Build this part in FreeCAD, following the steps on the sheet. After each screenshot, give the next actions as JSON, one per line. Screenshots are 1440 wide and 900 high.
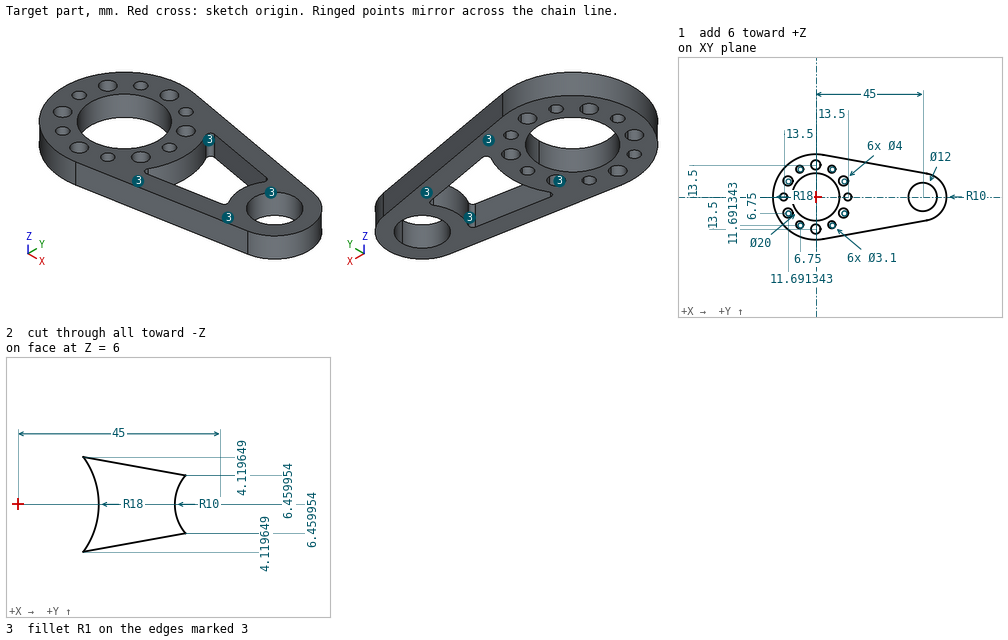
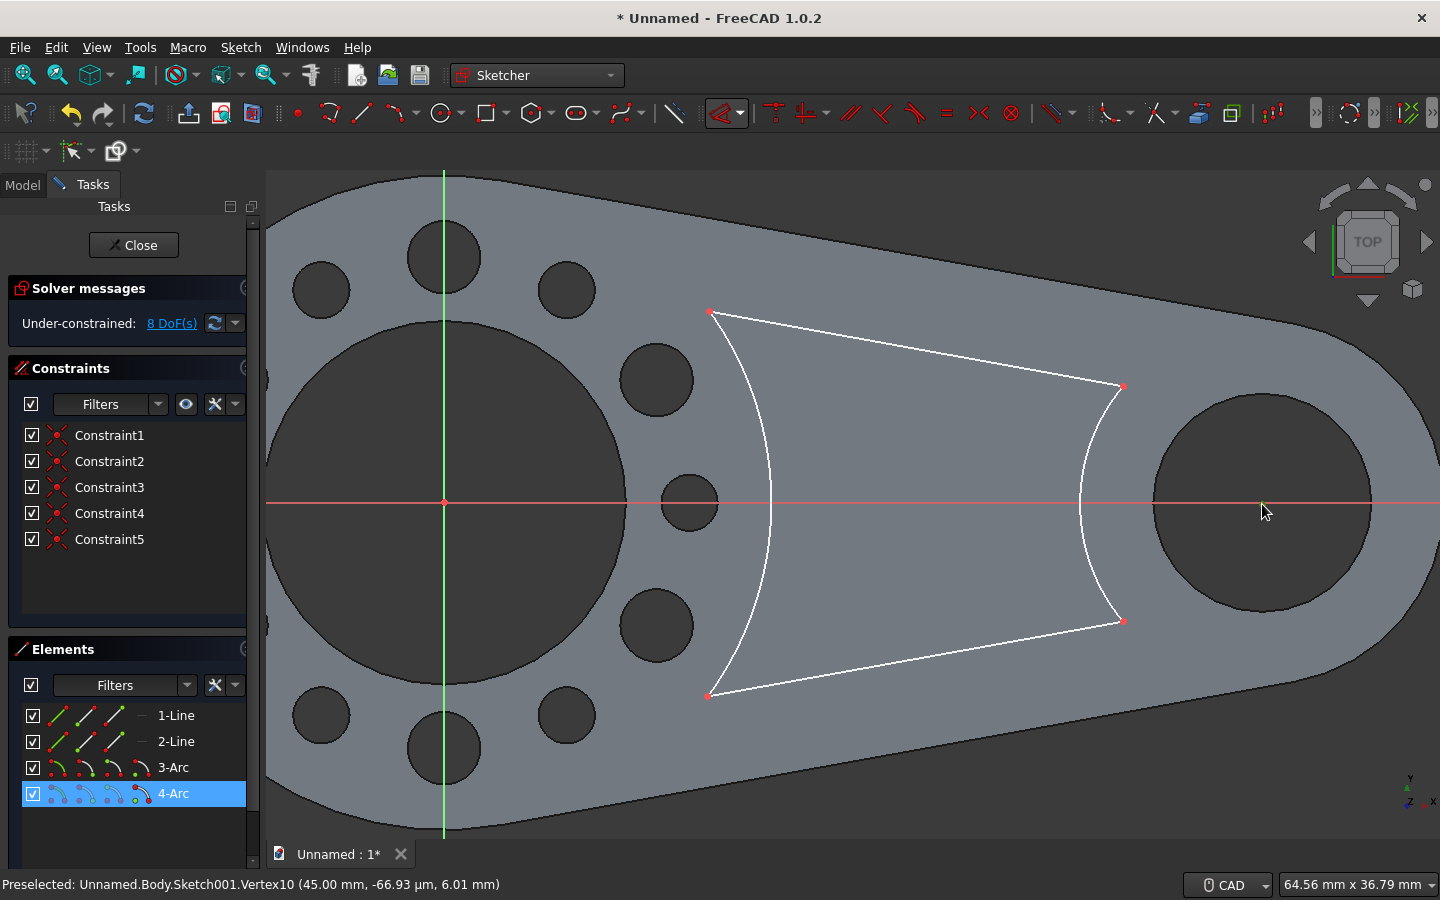
{"action": "left_click", "coordinate": [364, 503]}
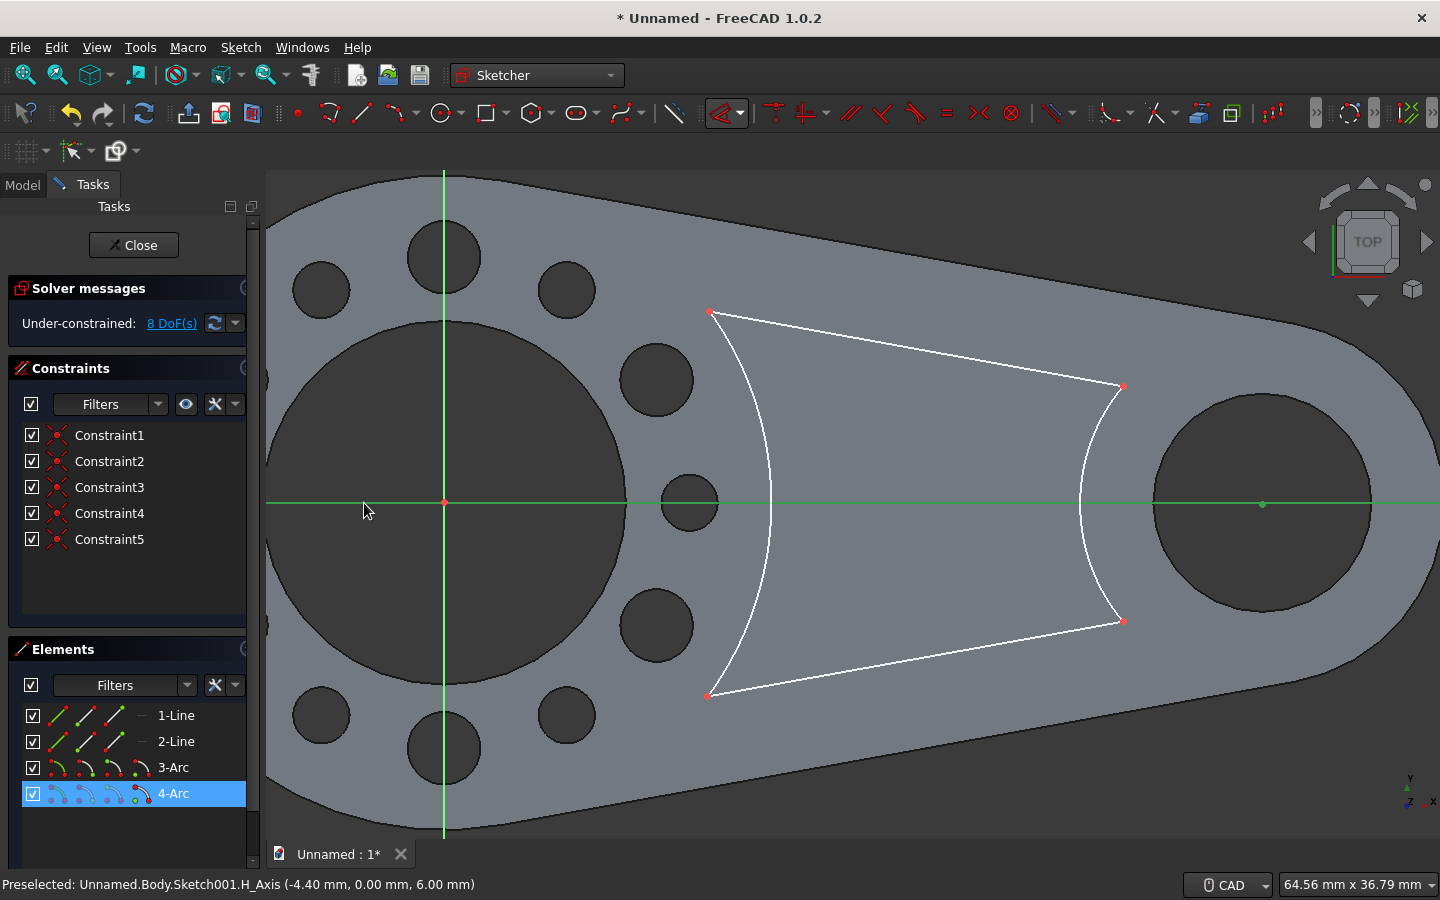
{"action": "key", "text": "c"}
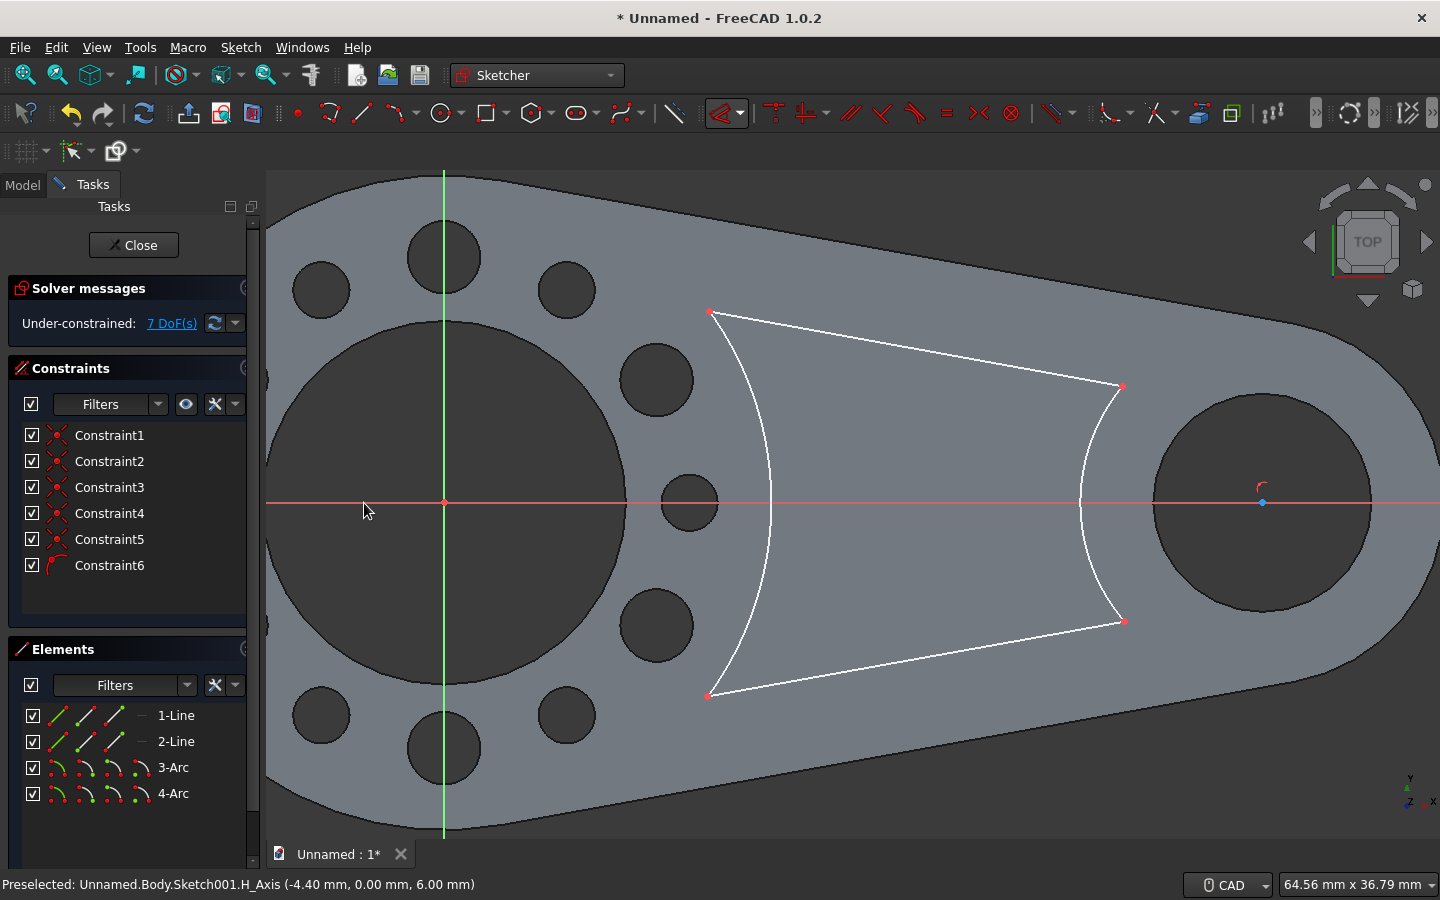
{"action": "left_click", "coordinate": [720, 114]}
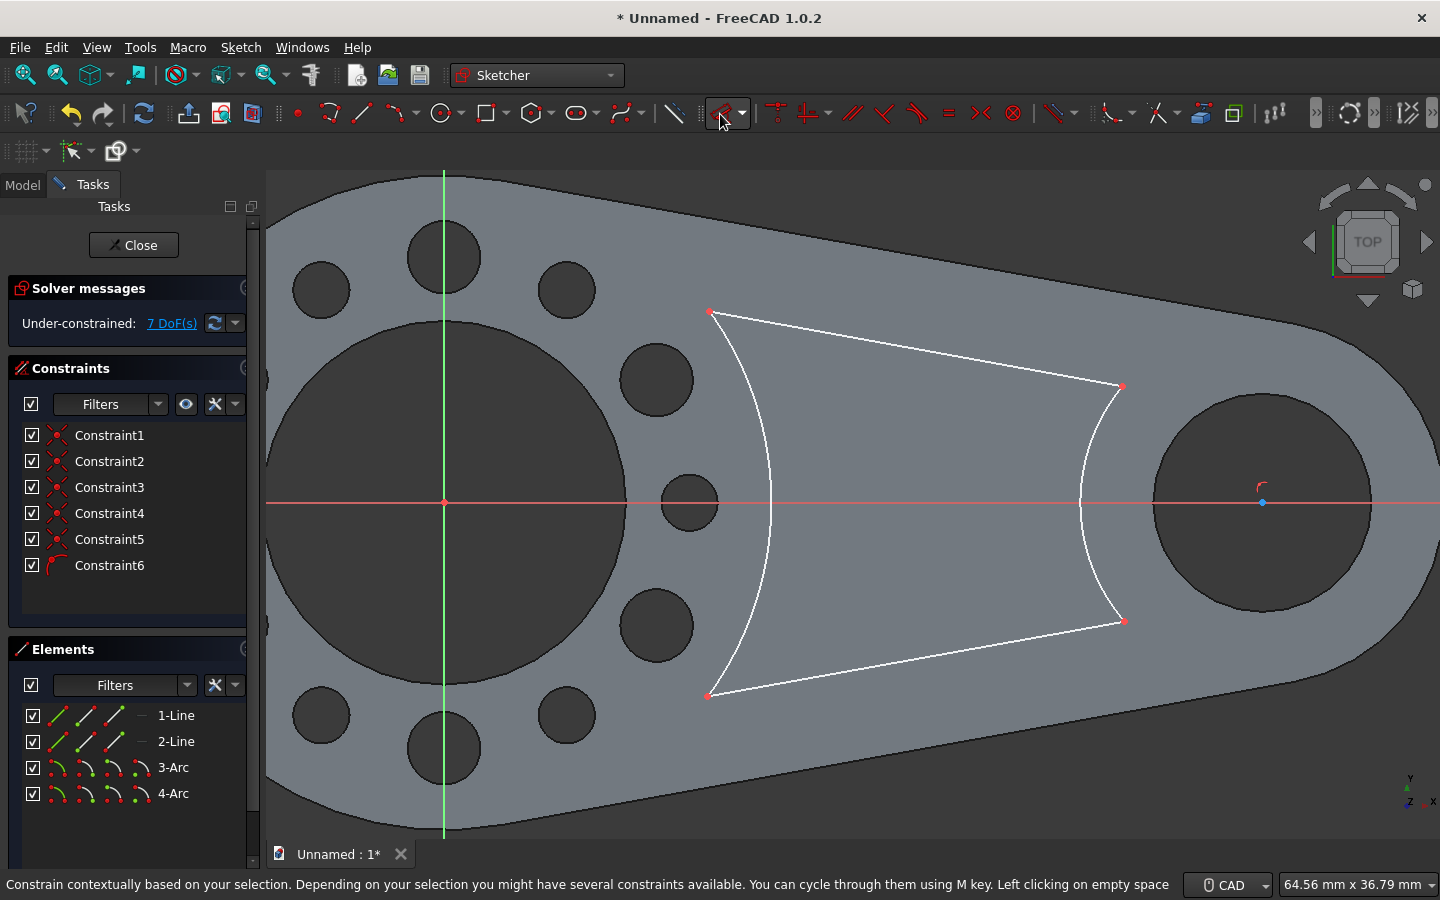
{"action": "left_click", "coordinate": [761, 586]}
{"action": "left_click", "coordinate": [792, 594]}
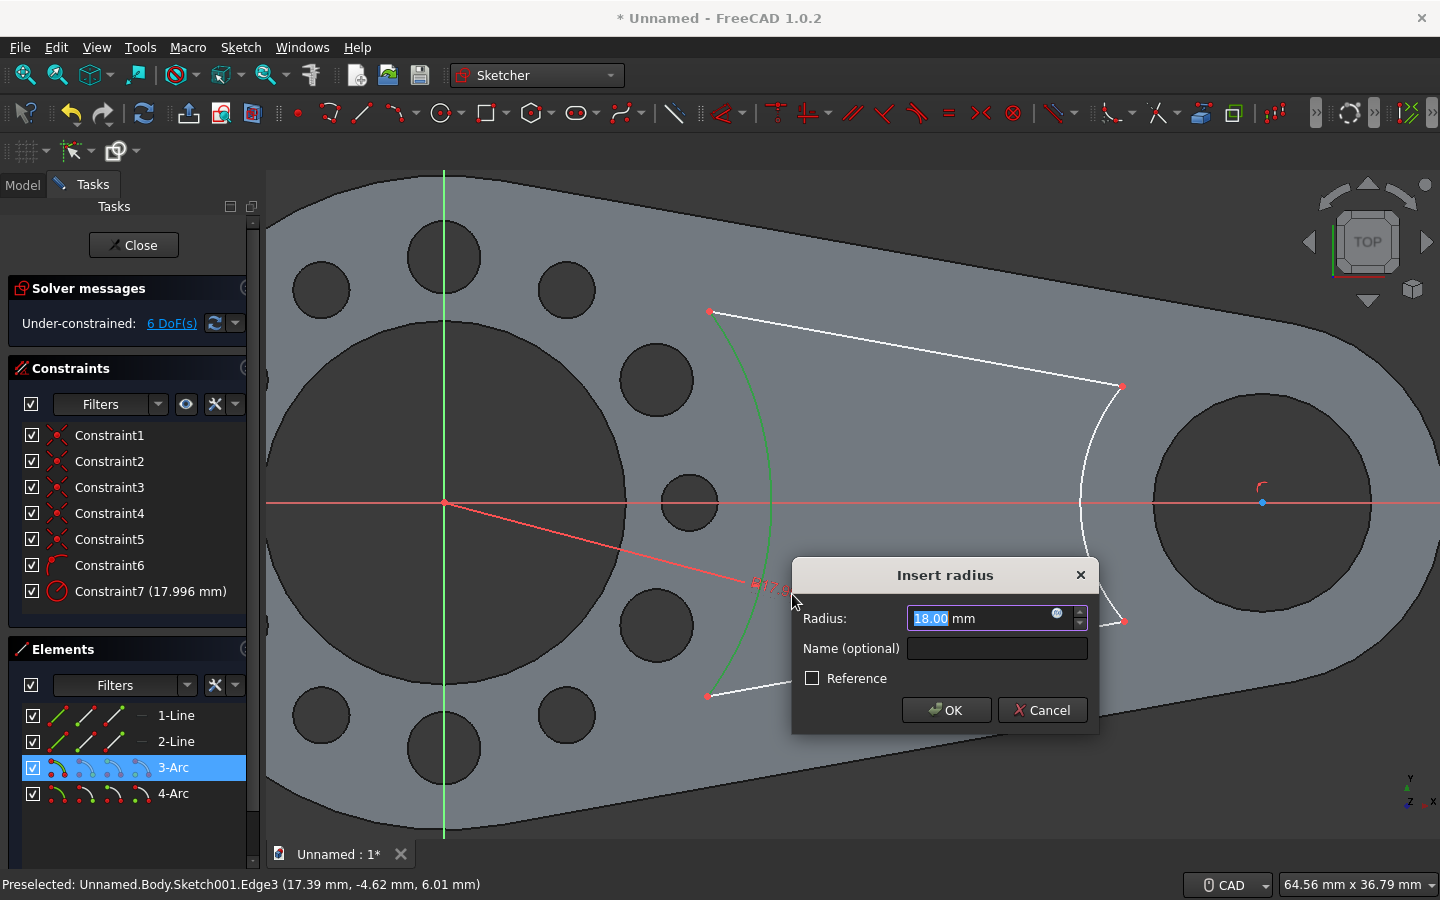
{"action": "type", "text": "18"}
{"action": "key", "text": "Return"}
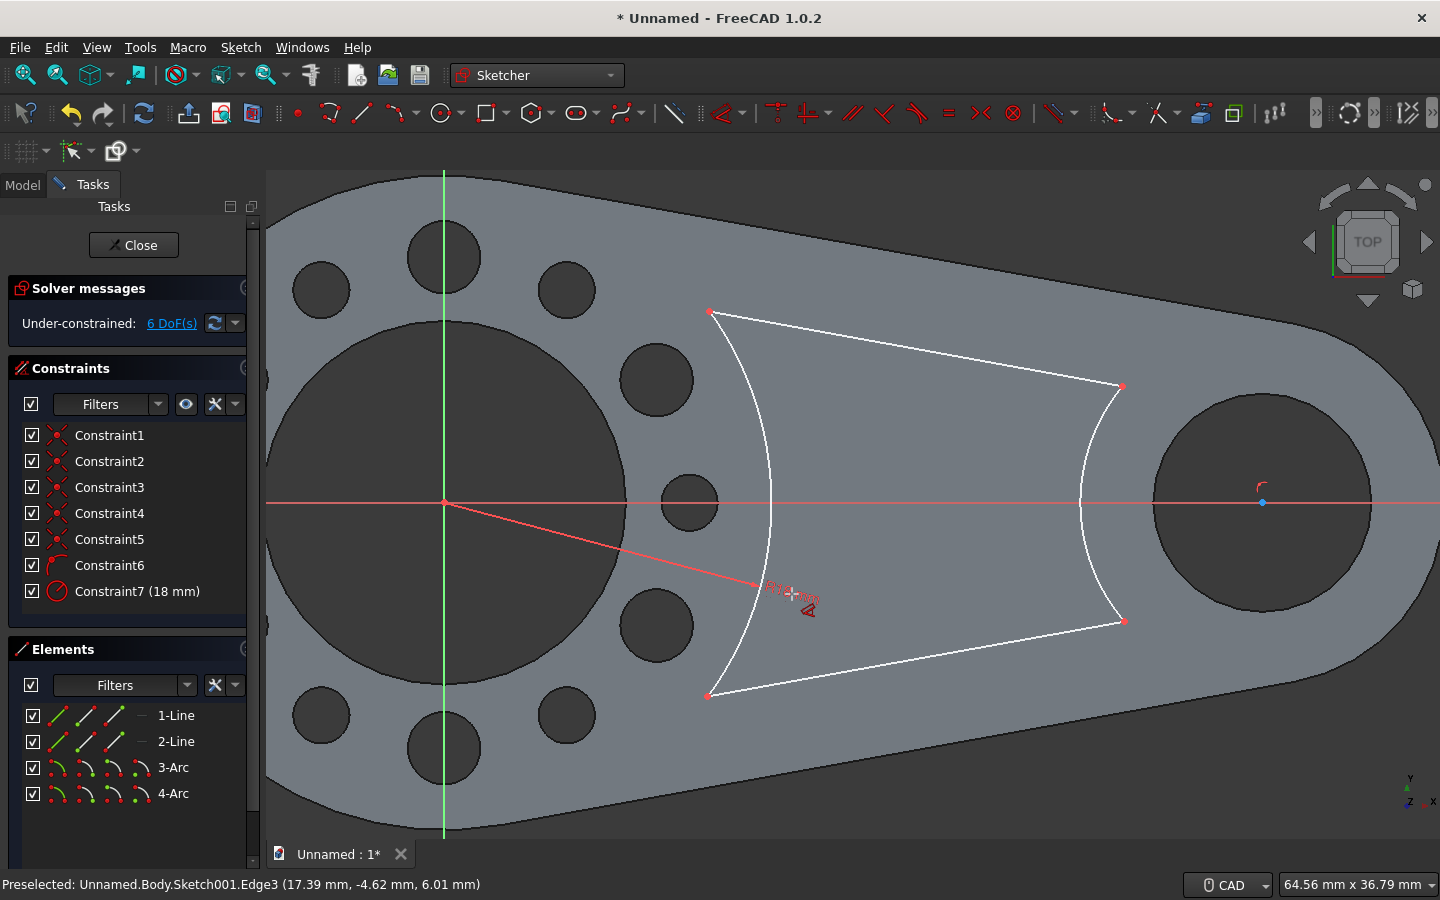
{"action": "left_click", "coordinate": [1087, 454]}
{"action": "left_click", "coordinate": [1056, 445]}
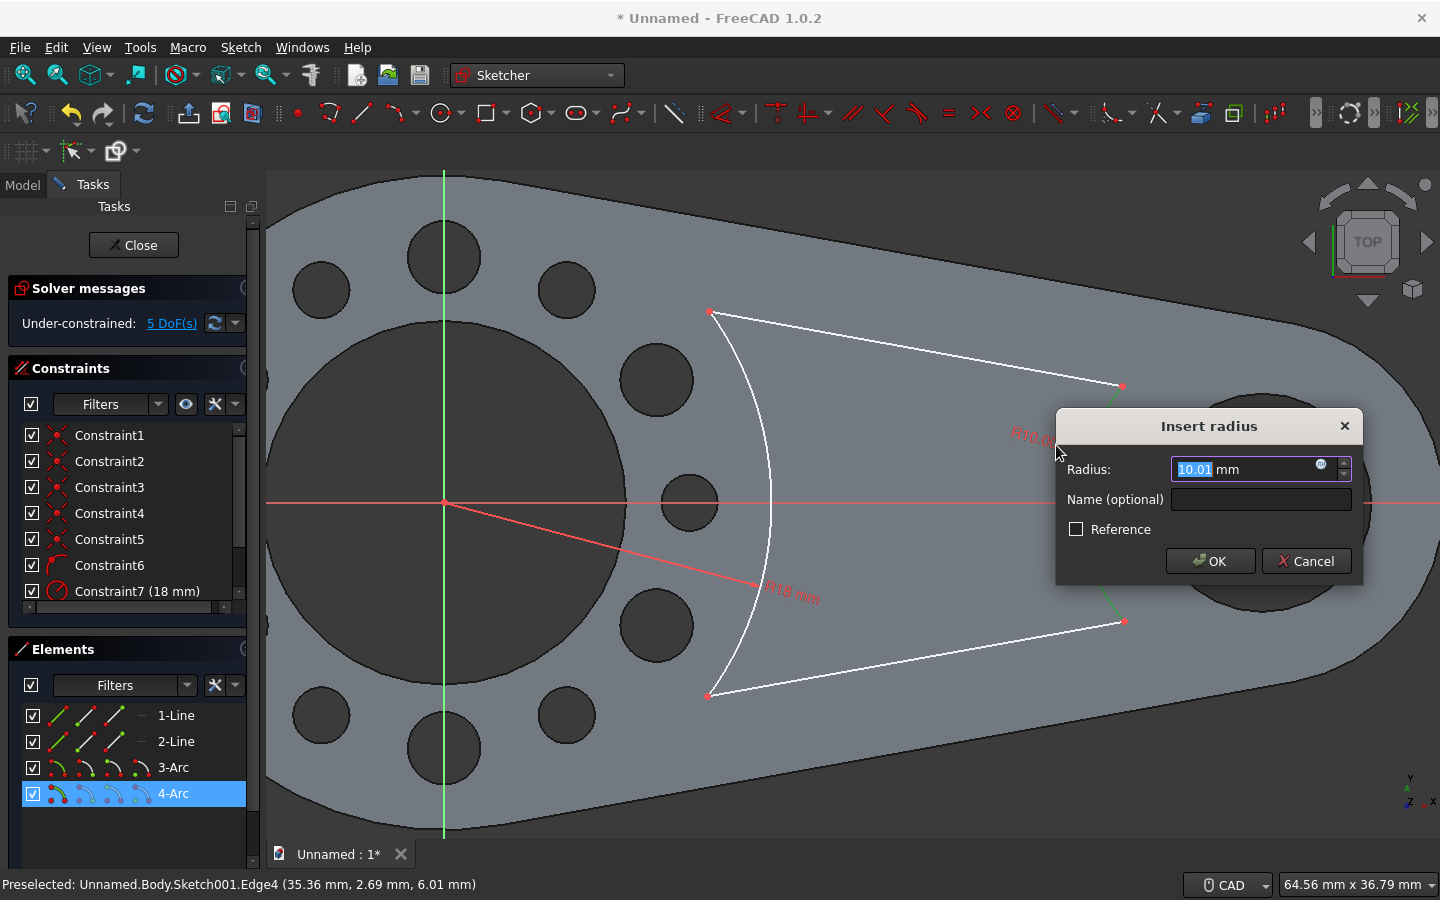
{"action": "type", "text": "10"}
{"action": "key", "text": "Return"}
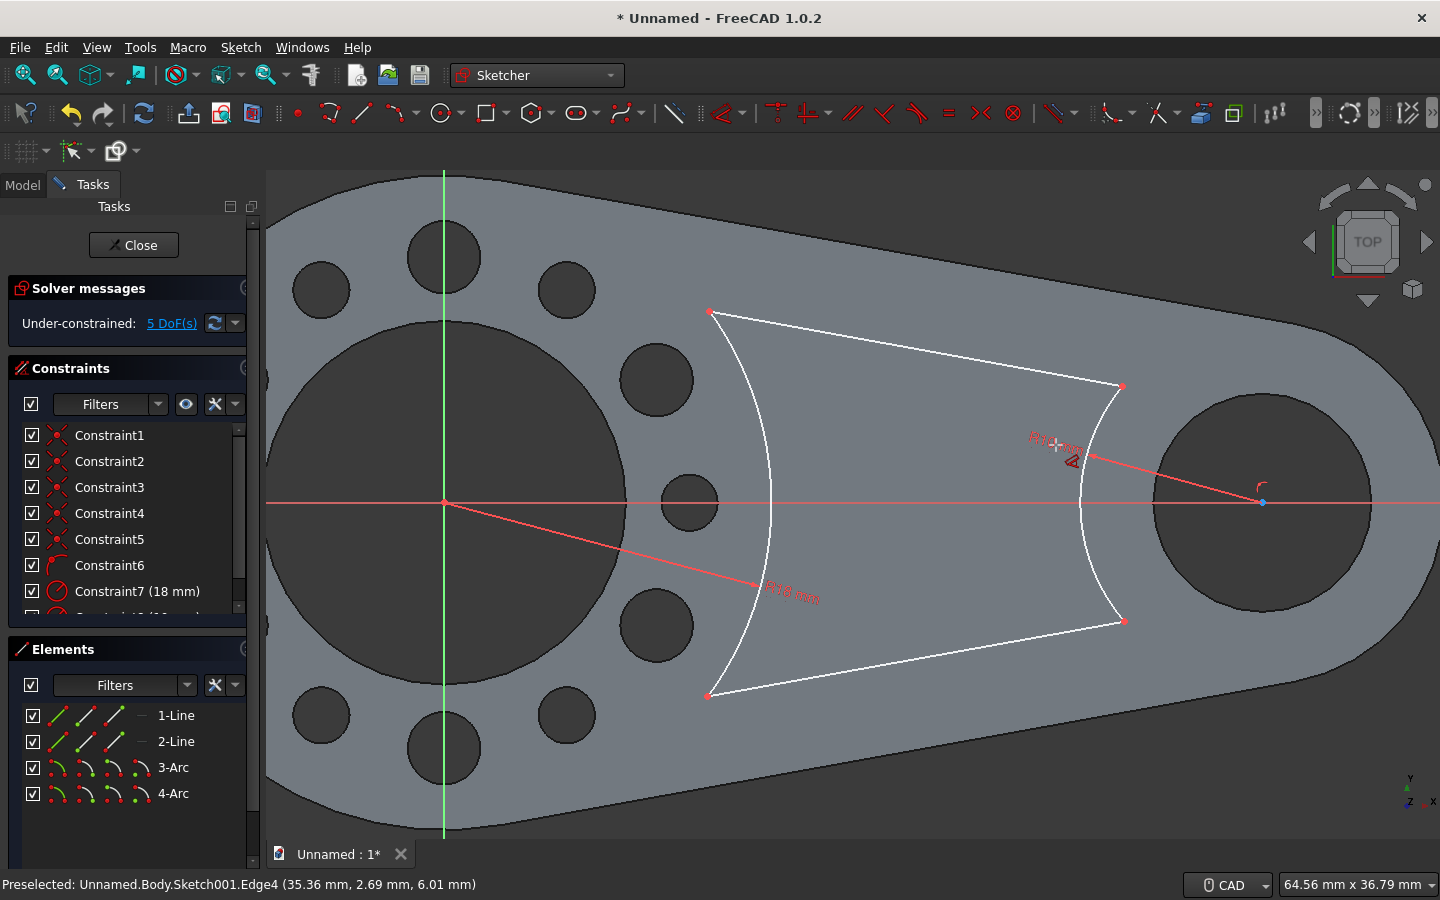
{"action": "left_click", "coordinate": [1262, 503]}
{"action": "left_click", "coordinate": [853, 537]}